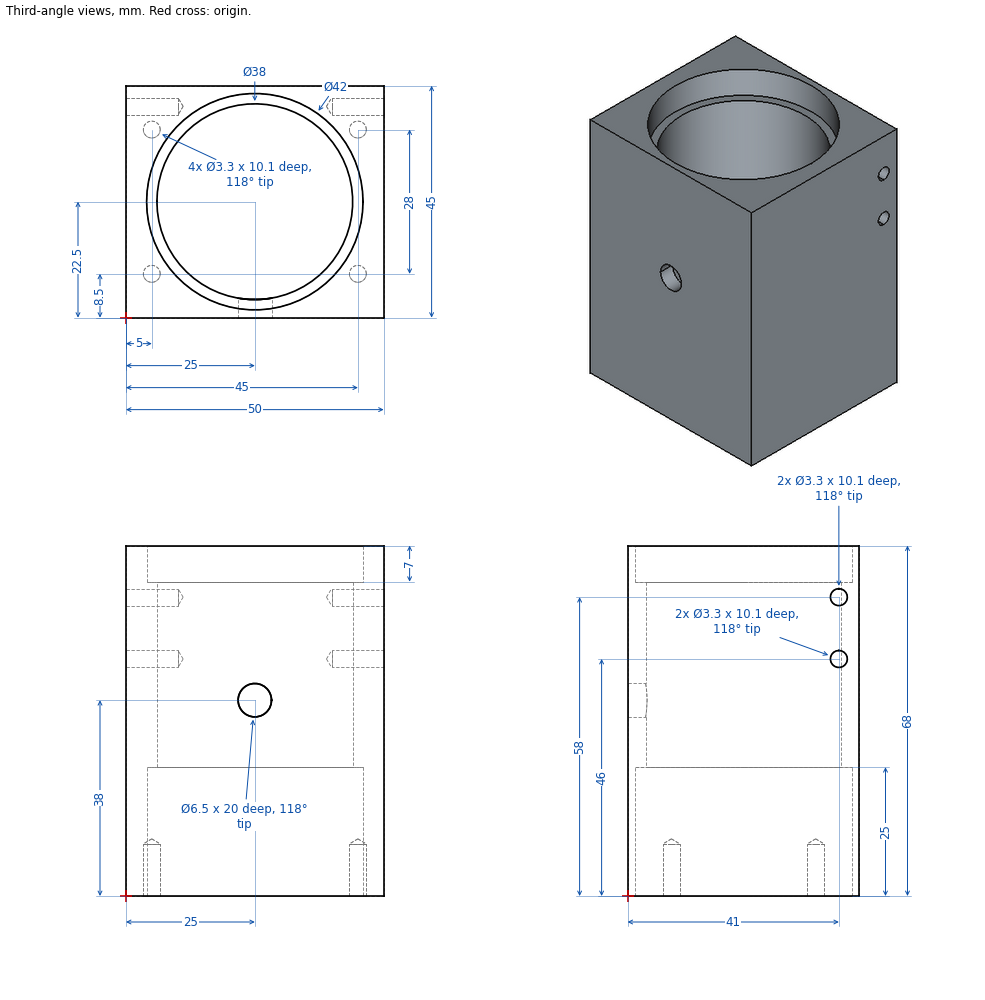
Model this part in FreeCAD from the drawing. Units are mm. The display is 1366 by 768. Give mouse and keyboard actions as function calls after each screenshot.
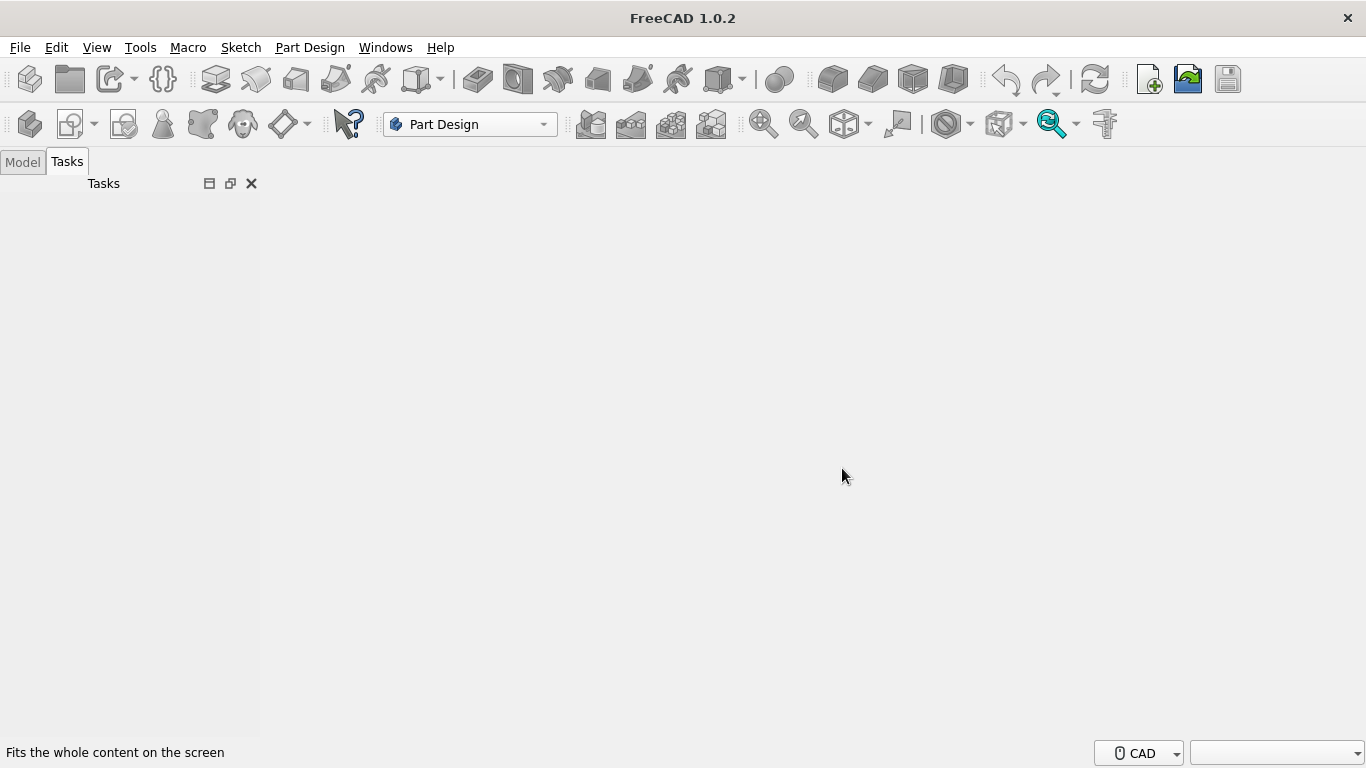
click(1148, 80)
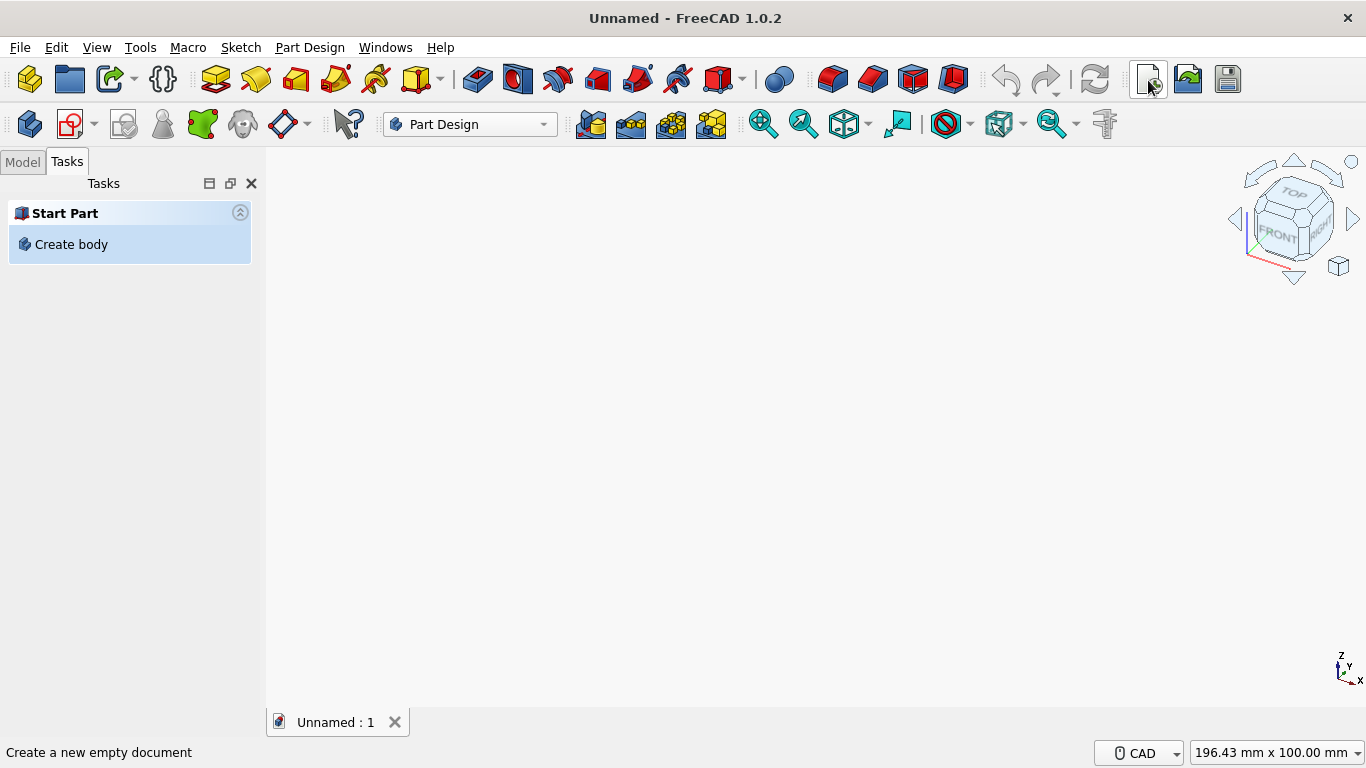
click(70, 124)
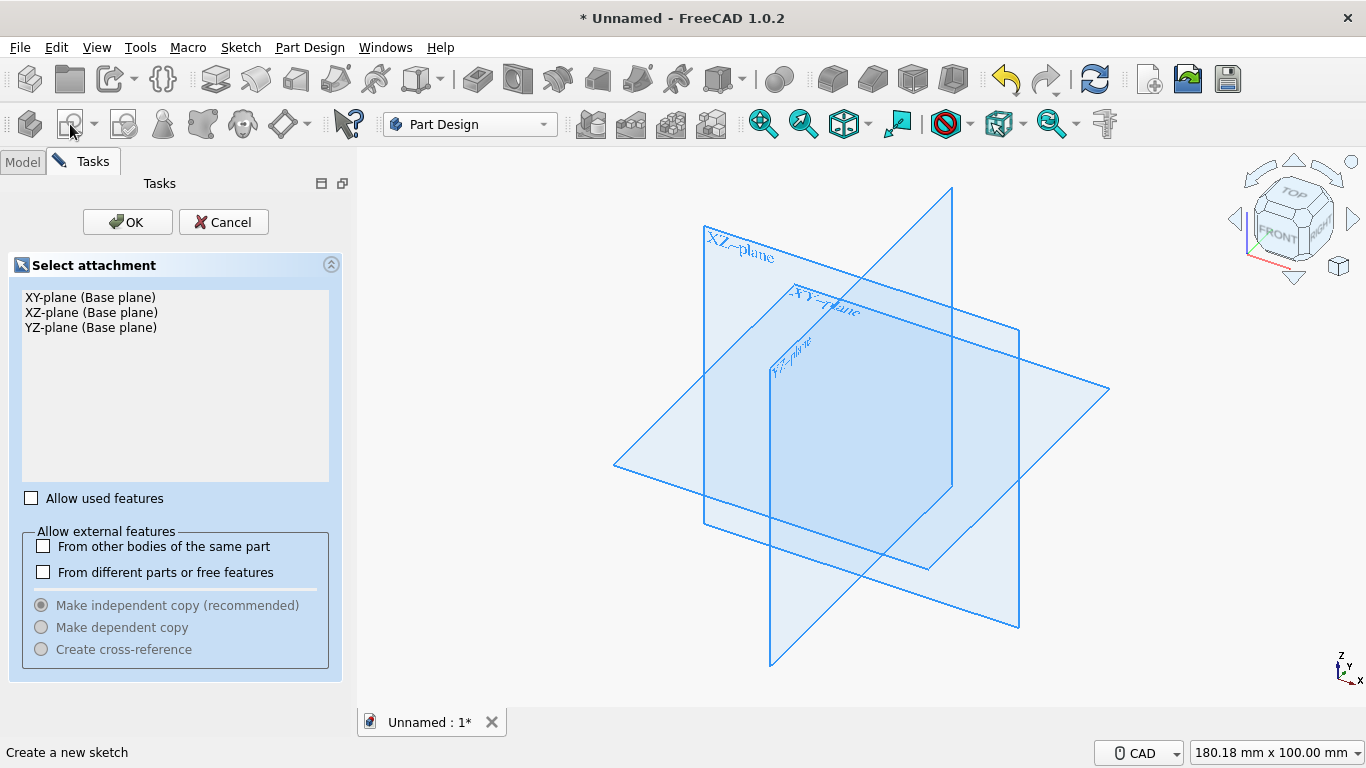
click(82, 298)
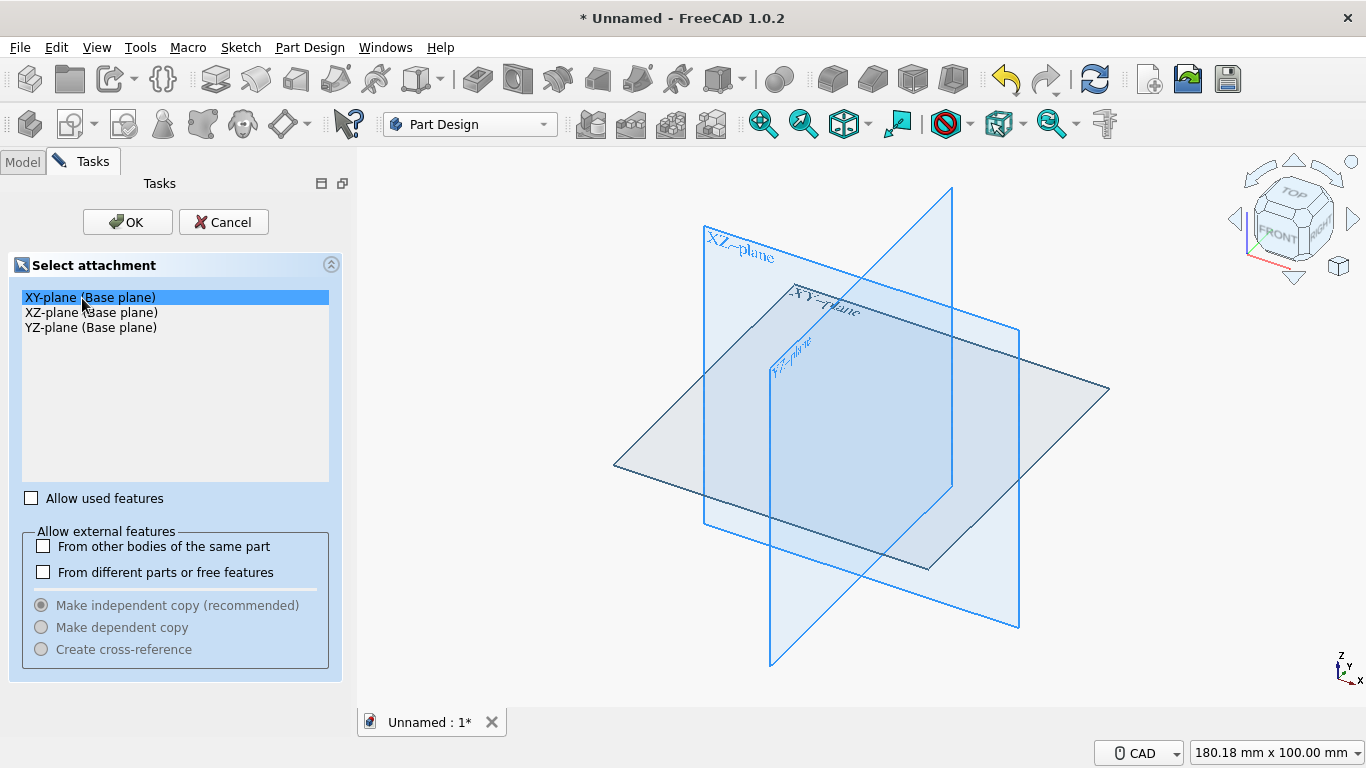
click(128, 222)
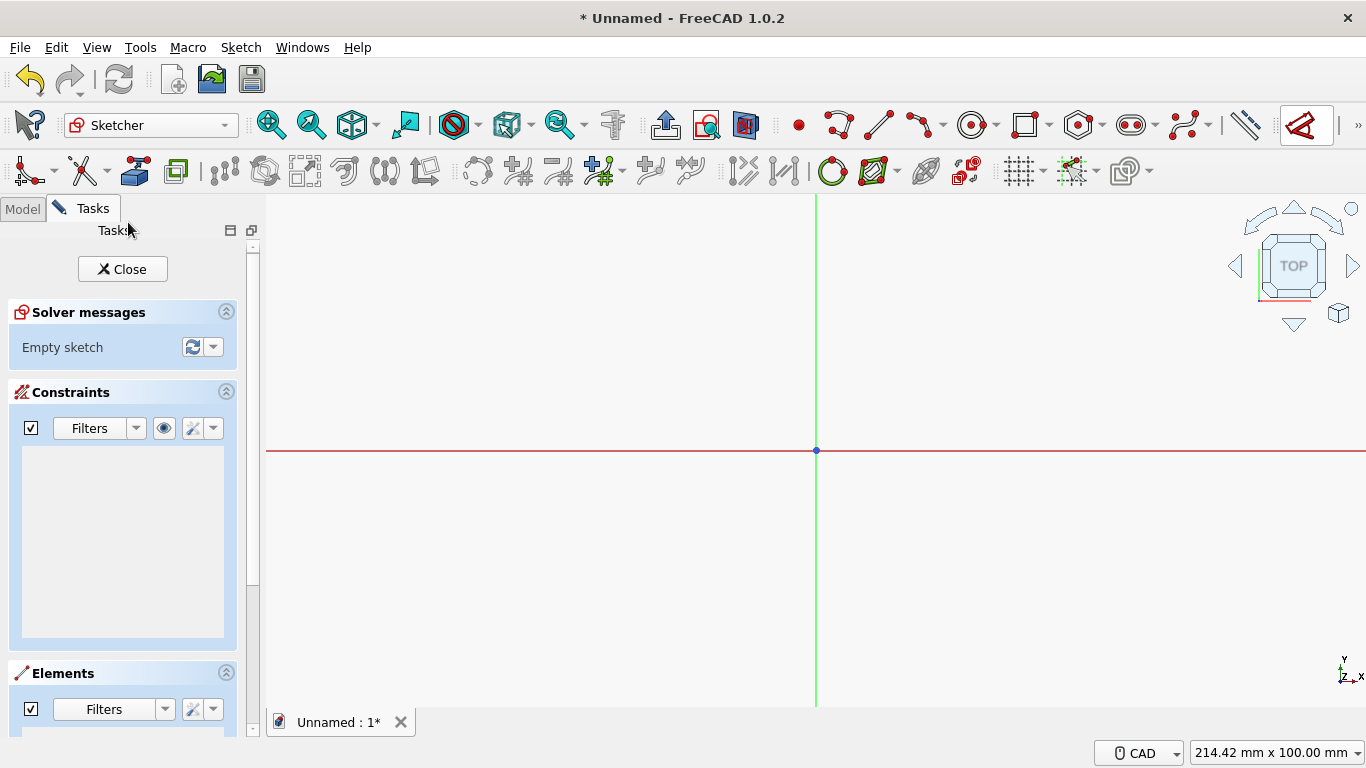
scroll(294, 679, down, 1)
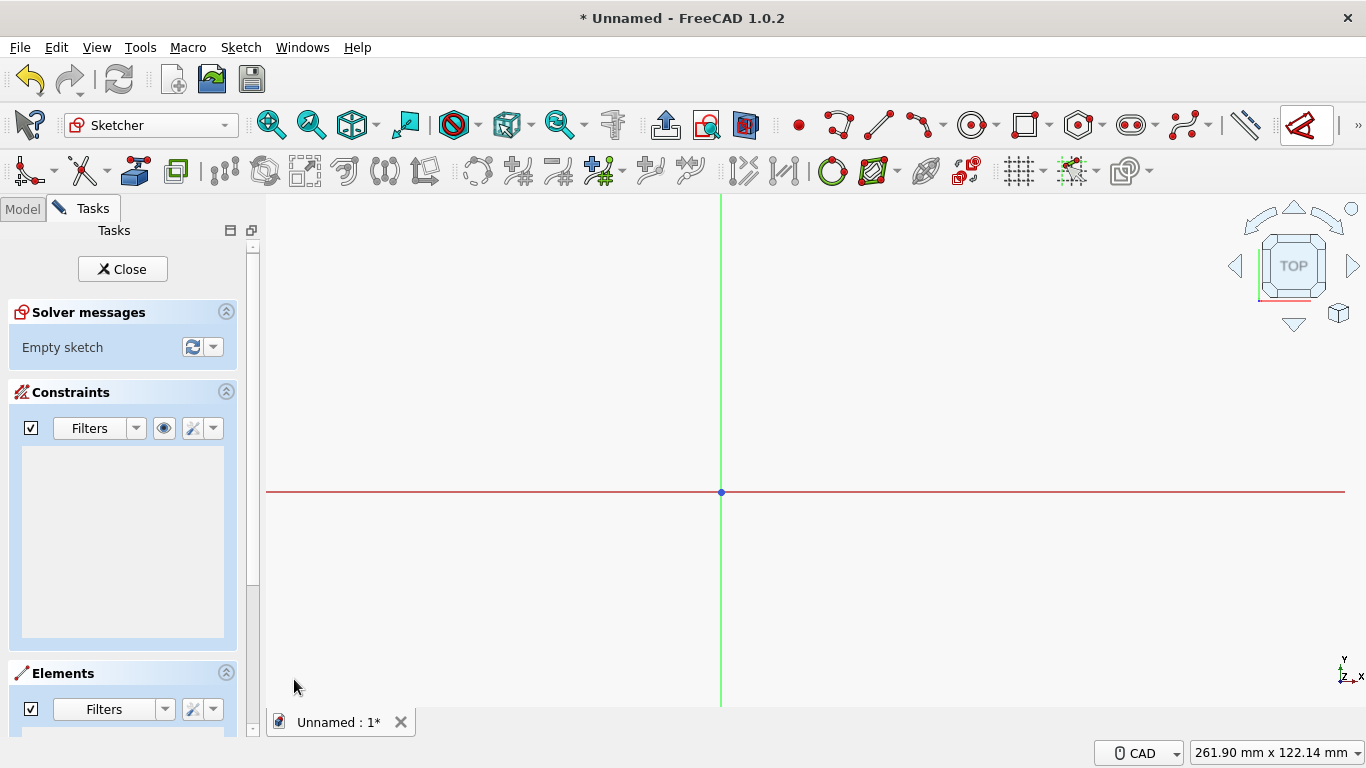
scroll(922, 333, up, 3)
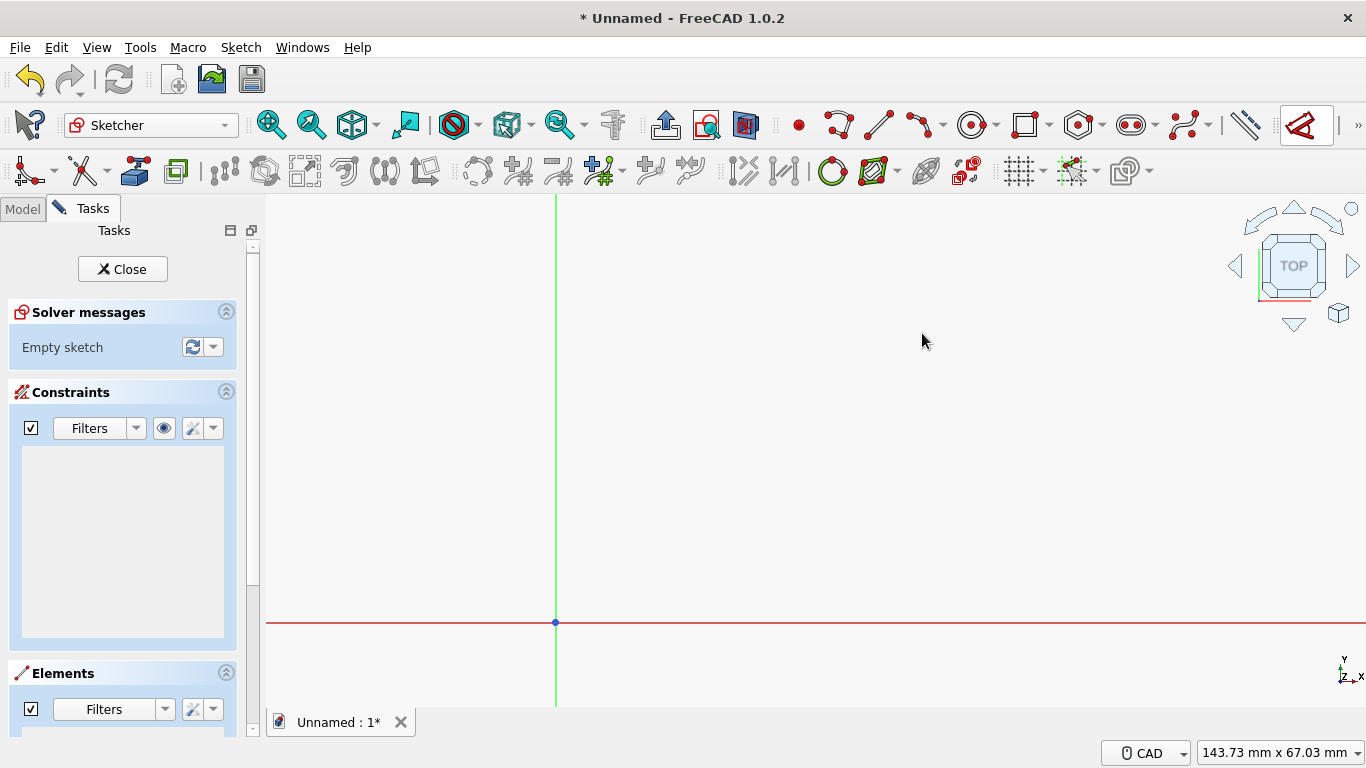
click(1026, 126)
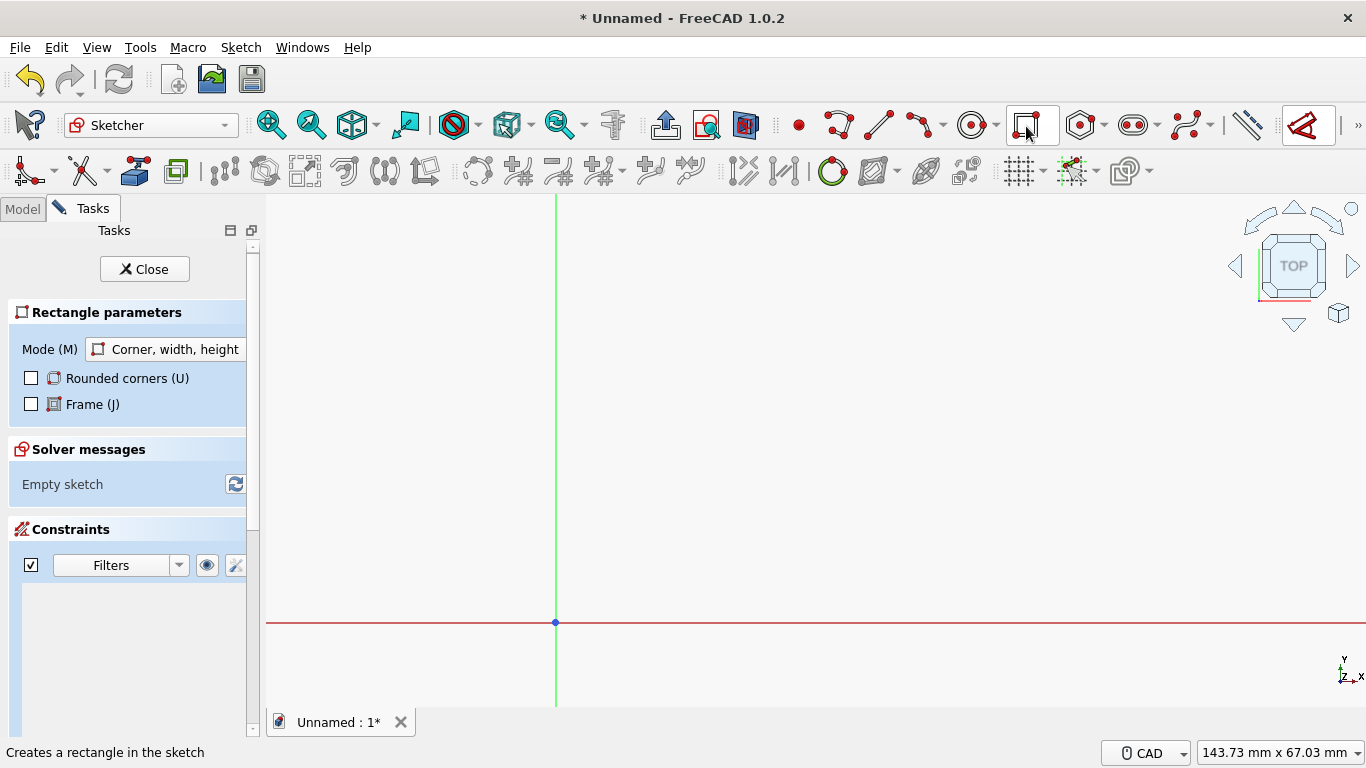
click(556, 623)
move(939, 278)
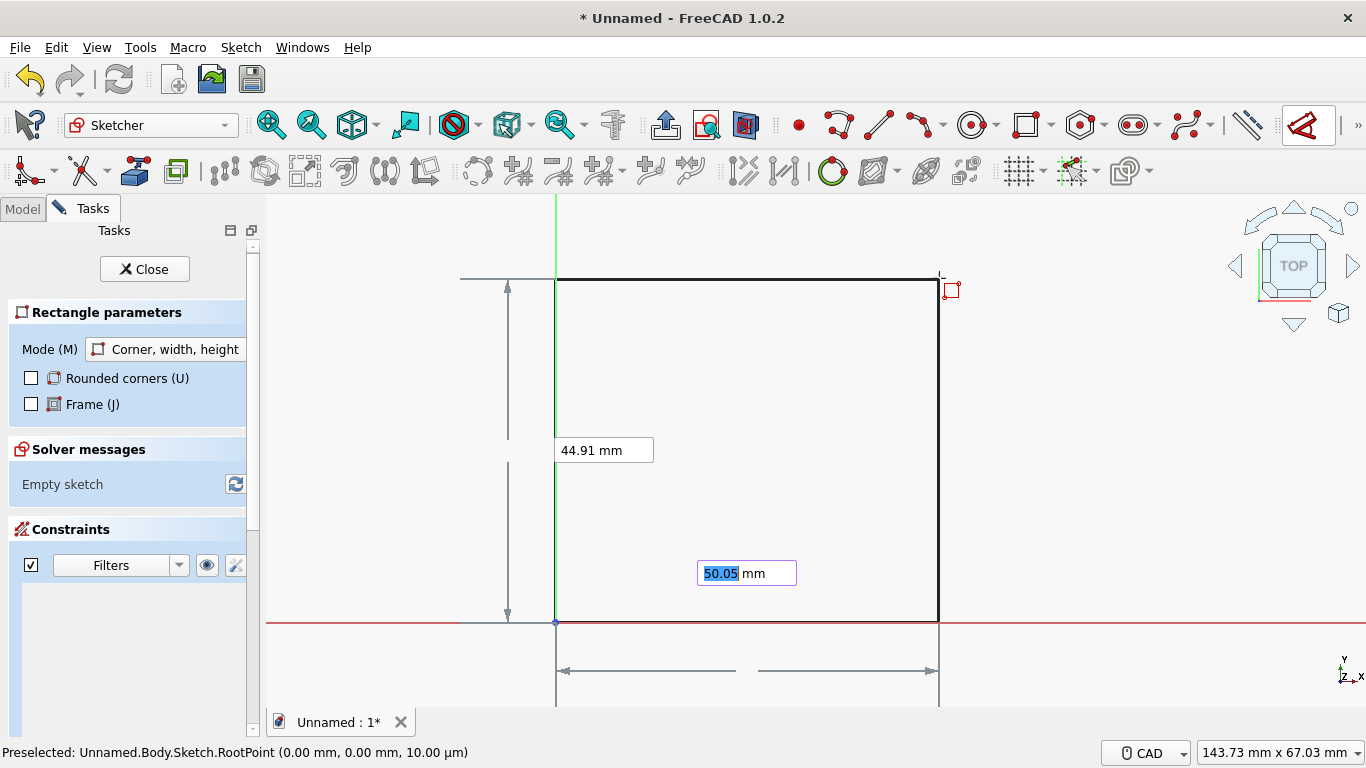
text(50)
key(Tab)
text(45)
key(Return)
key(Escape)